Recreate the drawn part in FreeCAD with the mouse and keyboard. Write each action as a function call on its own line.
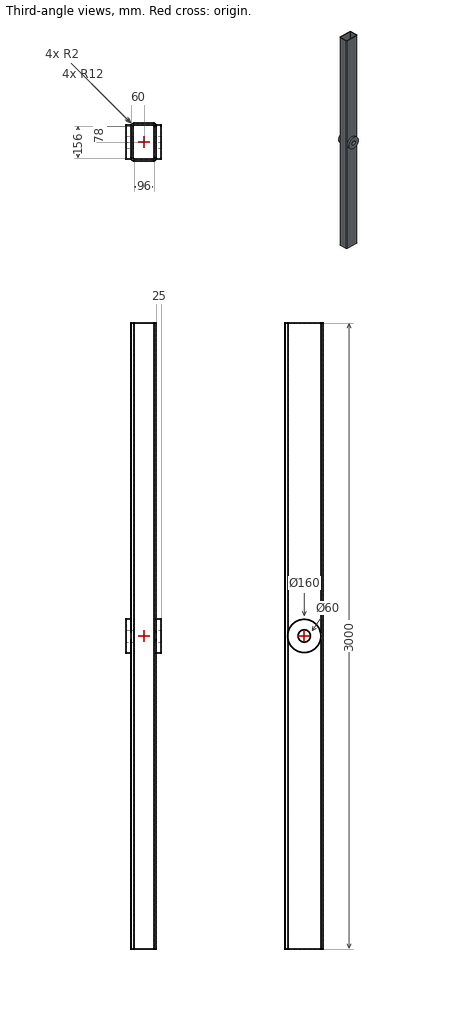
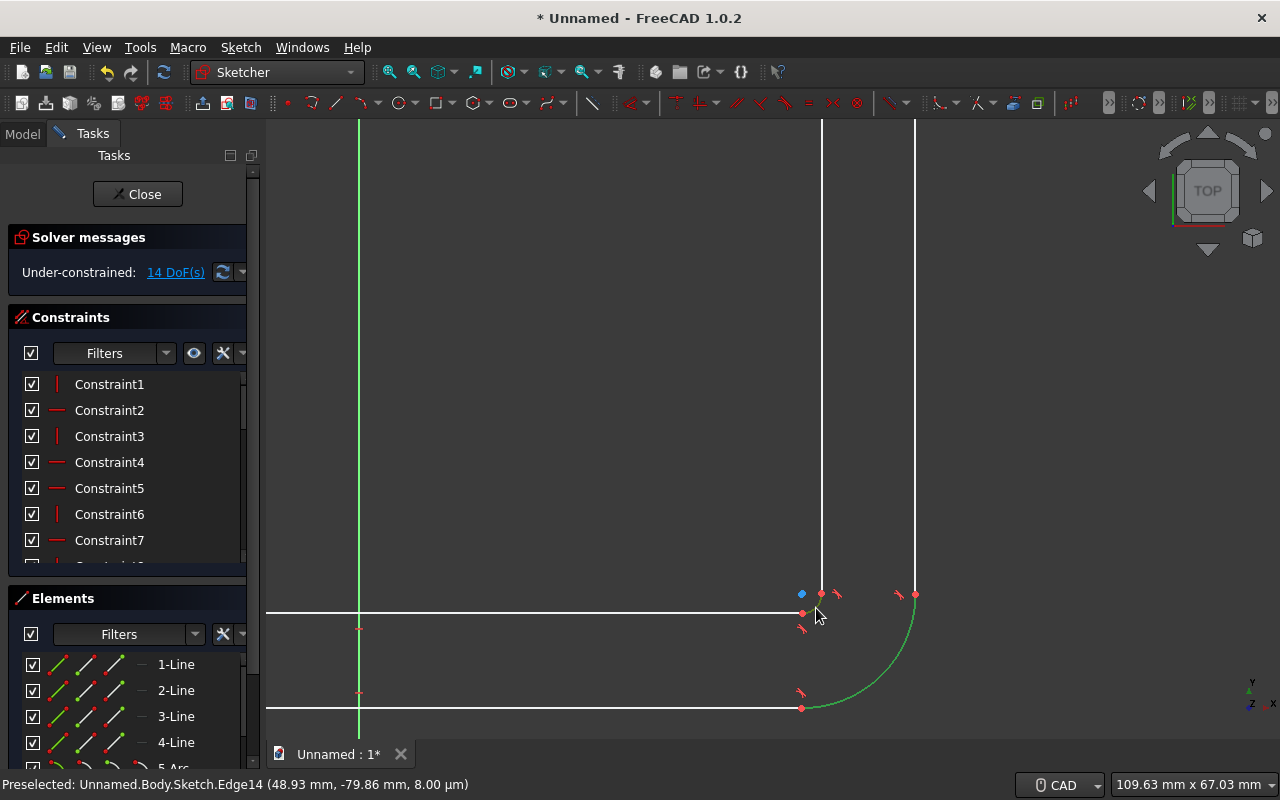
click(676, 104)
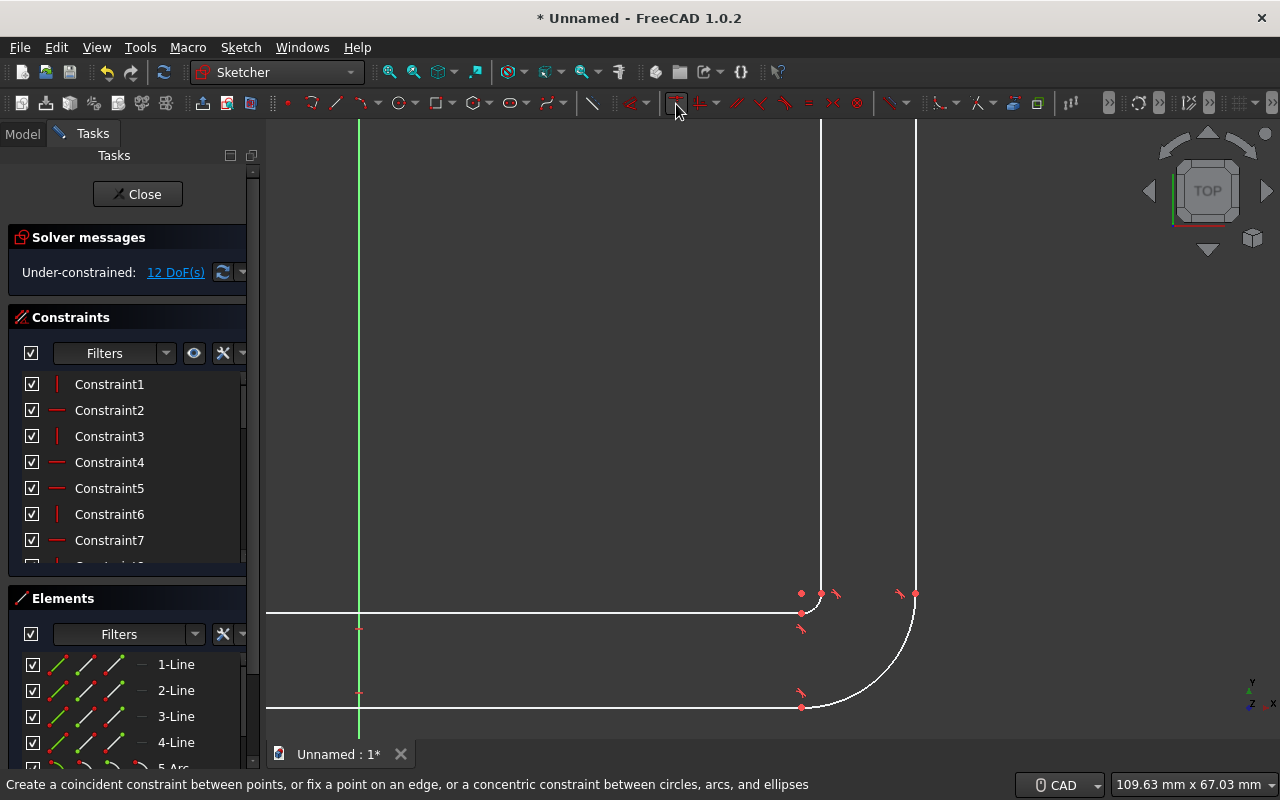
scroll(818, 611, down, 7)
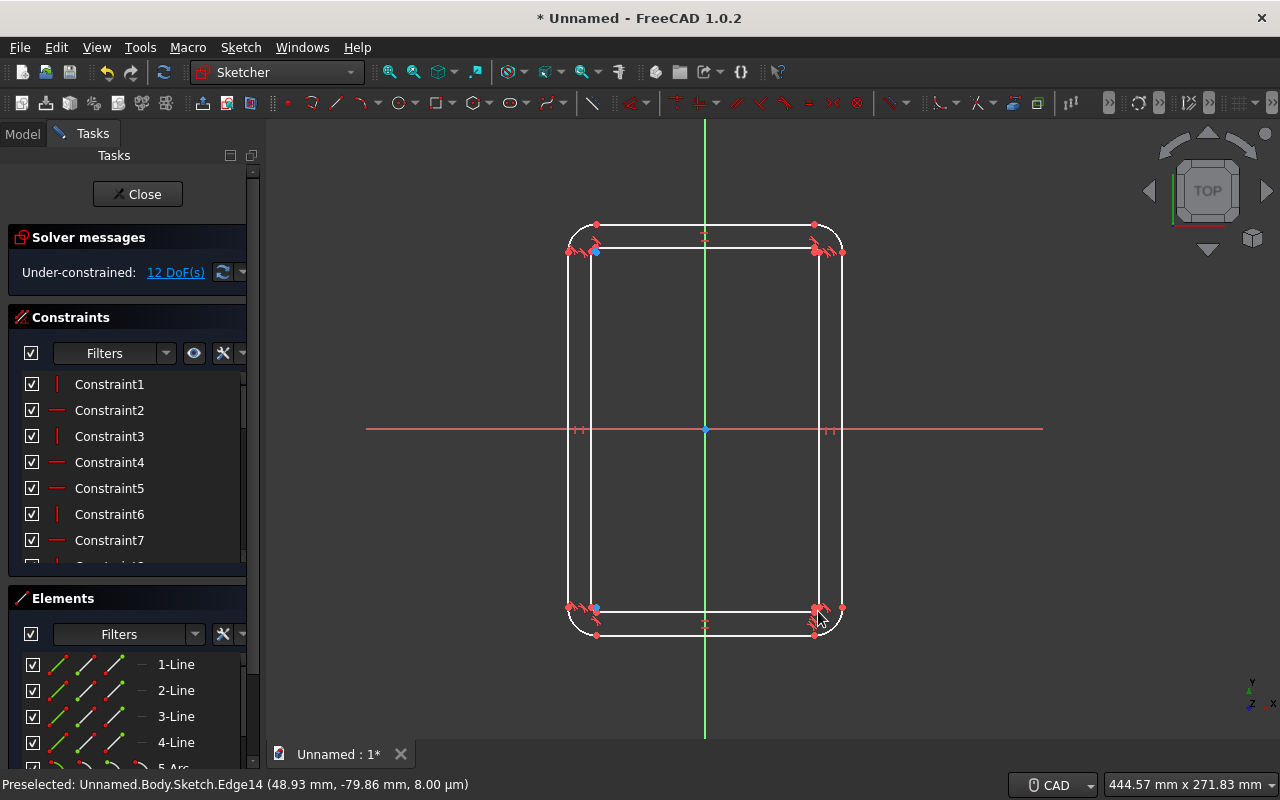
click(571, 620)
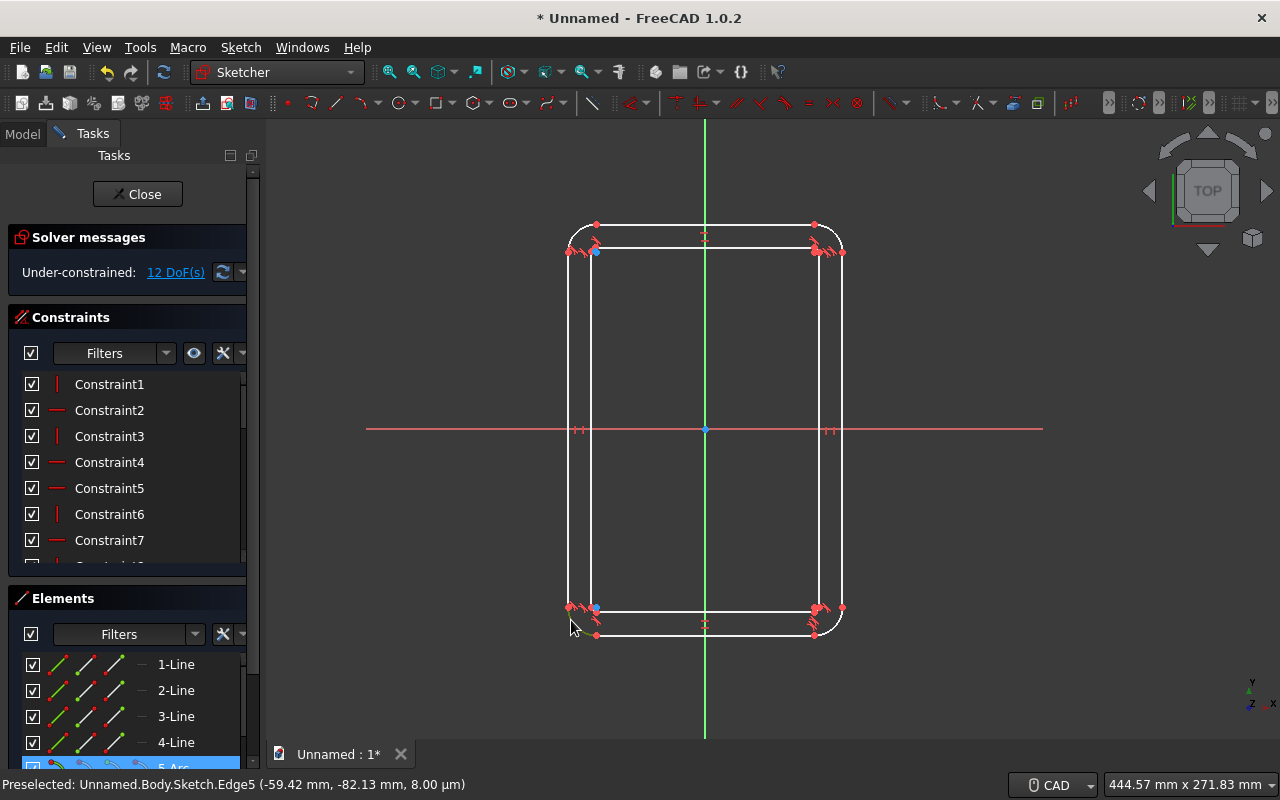
scroll(593, 611, up, 7)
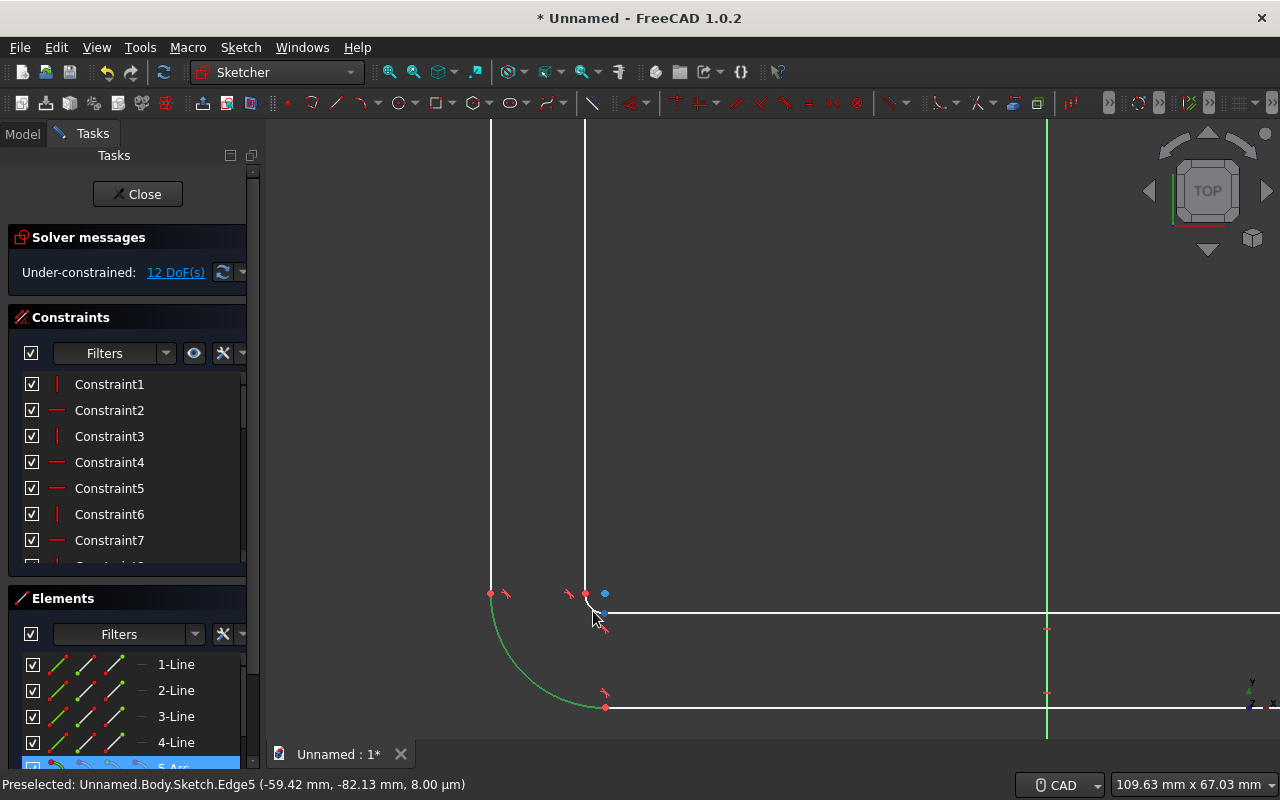
click(591, 608)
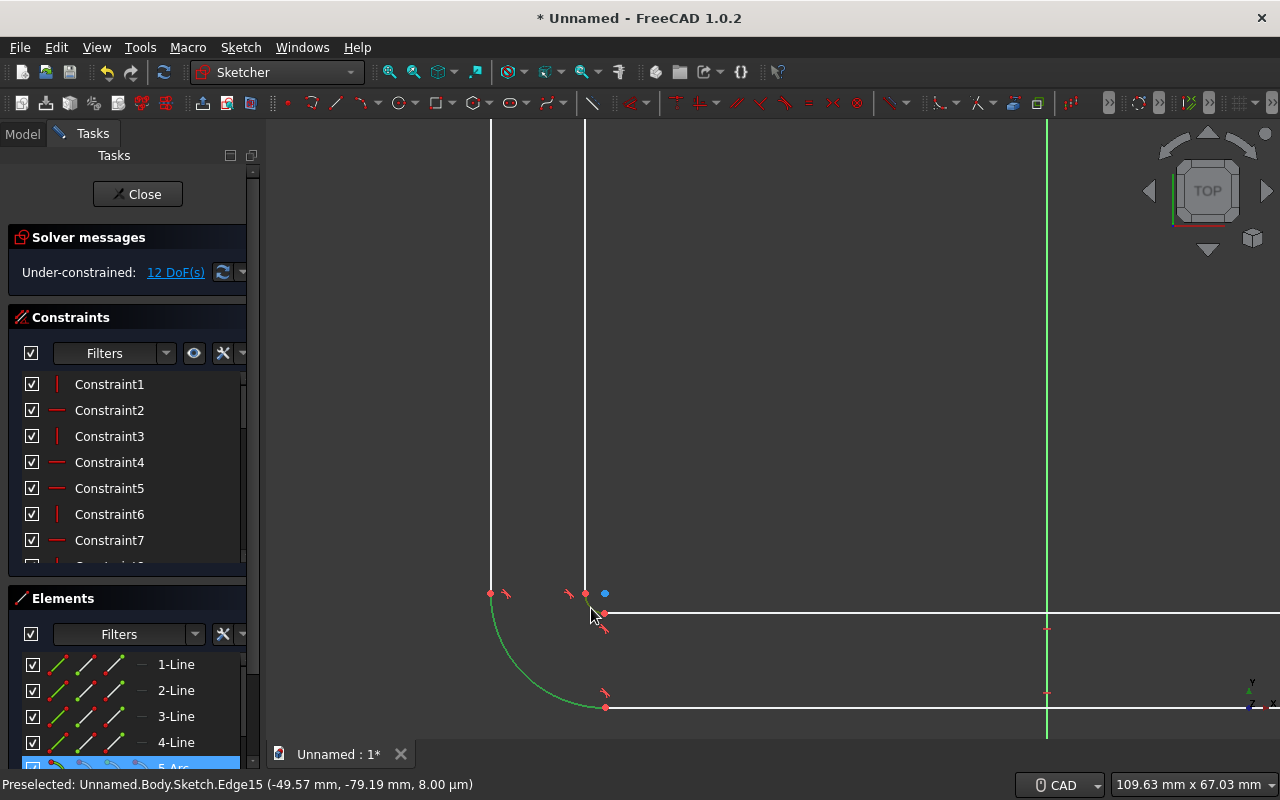
click(676, 104)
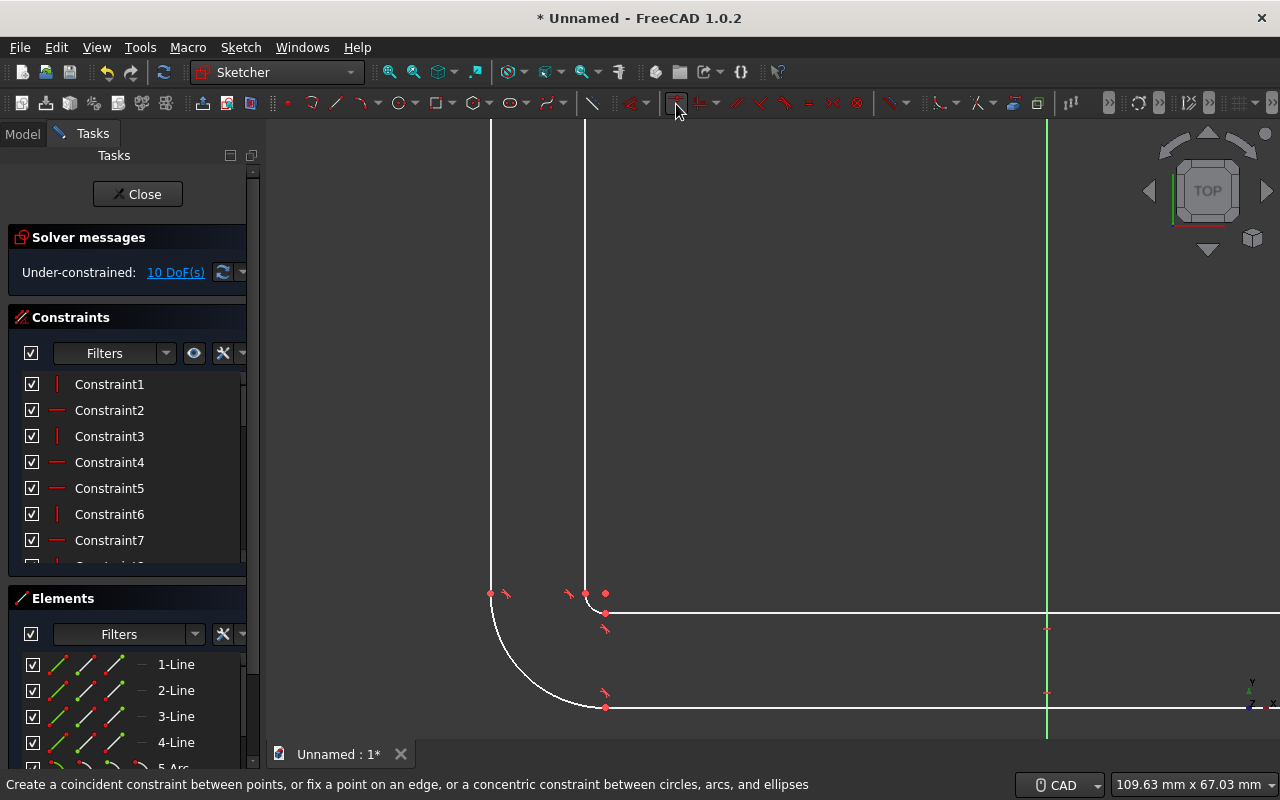
scroll(592, 611, down, 7)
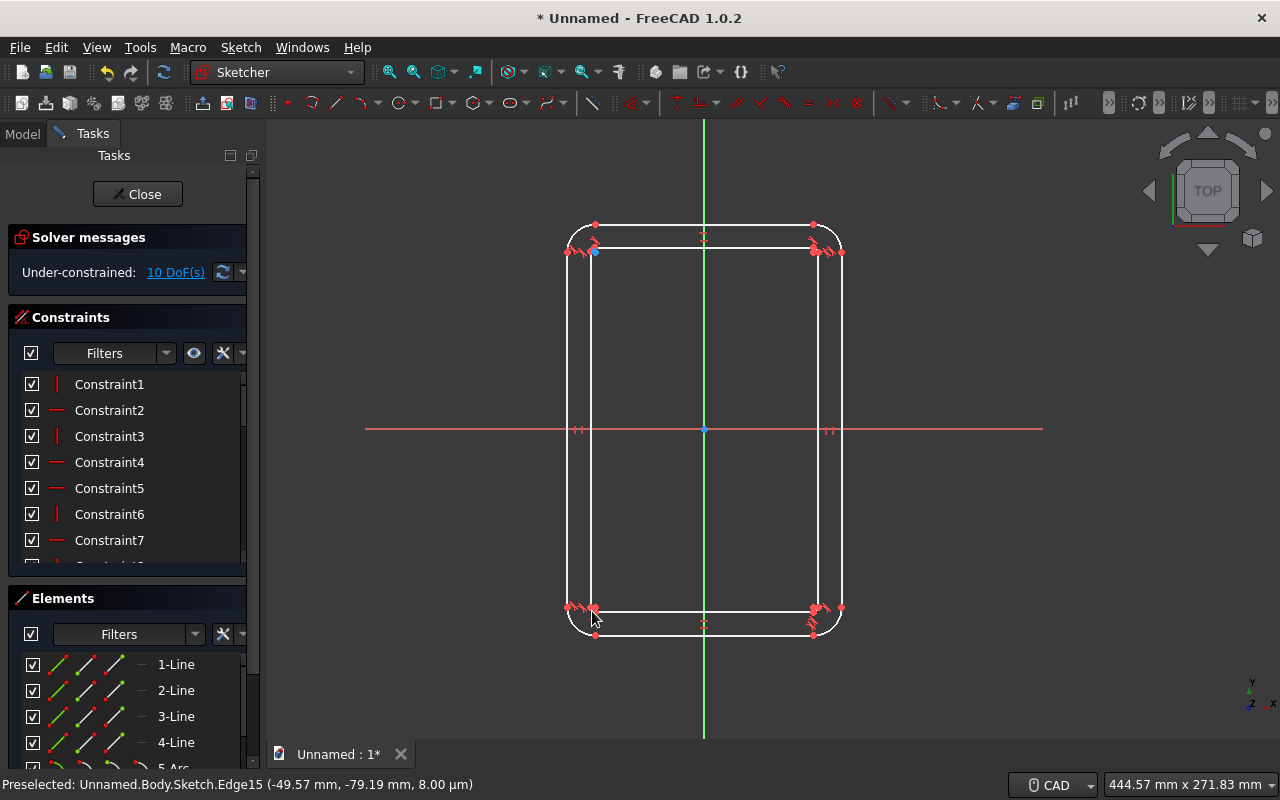
click(570, 620)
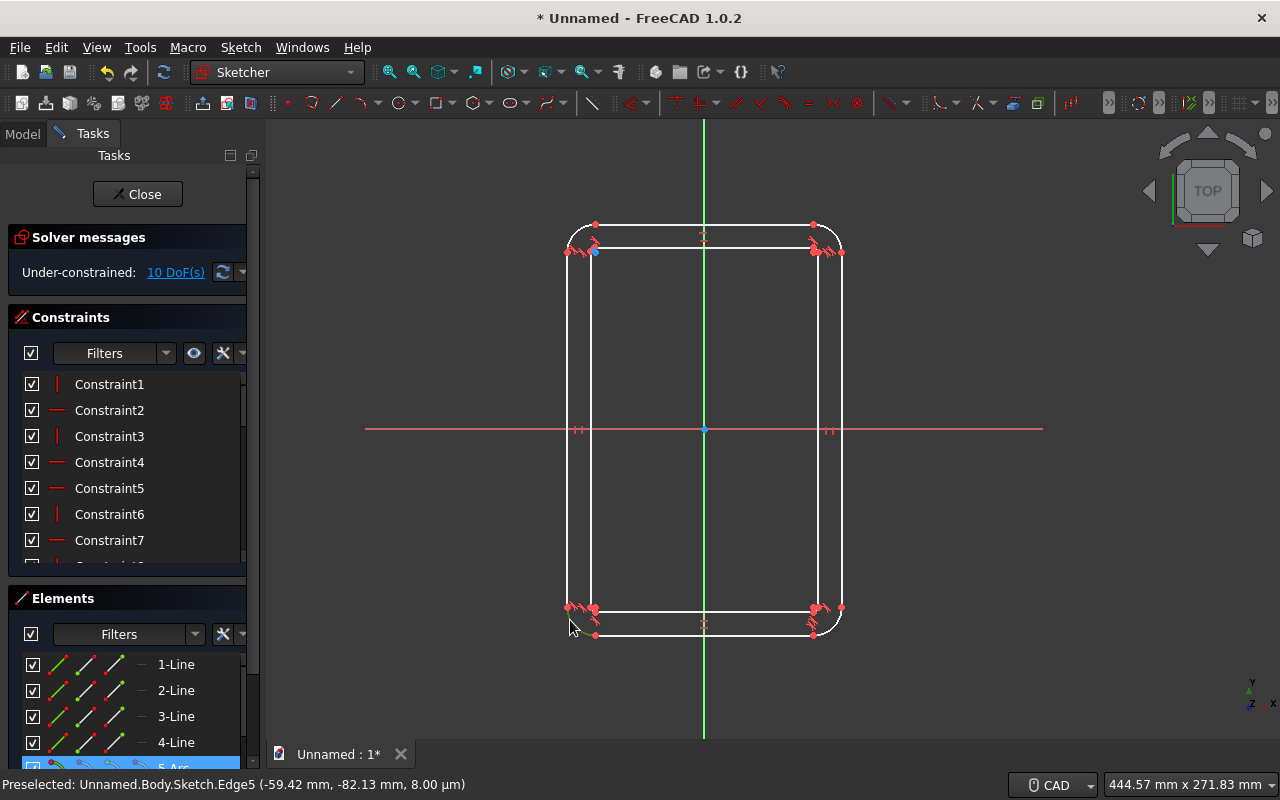
click(826, 632)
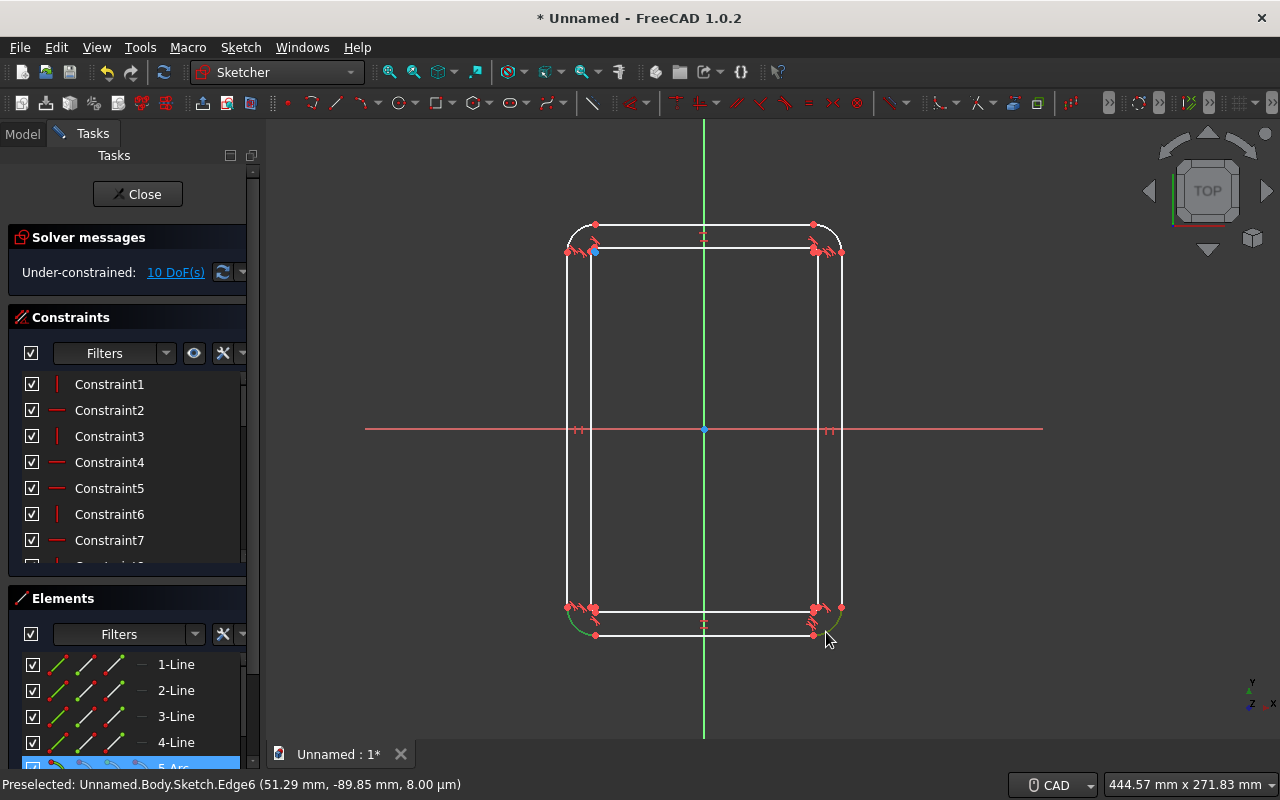
click(839, 240)